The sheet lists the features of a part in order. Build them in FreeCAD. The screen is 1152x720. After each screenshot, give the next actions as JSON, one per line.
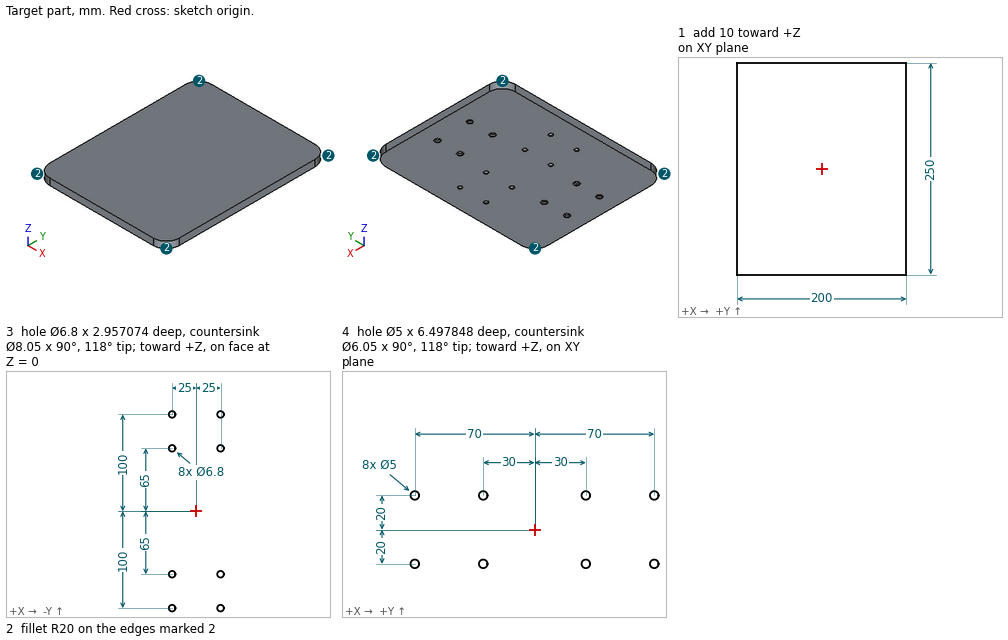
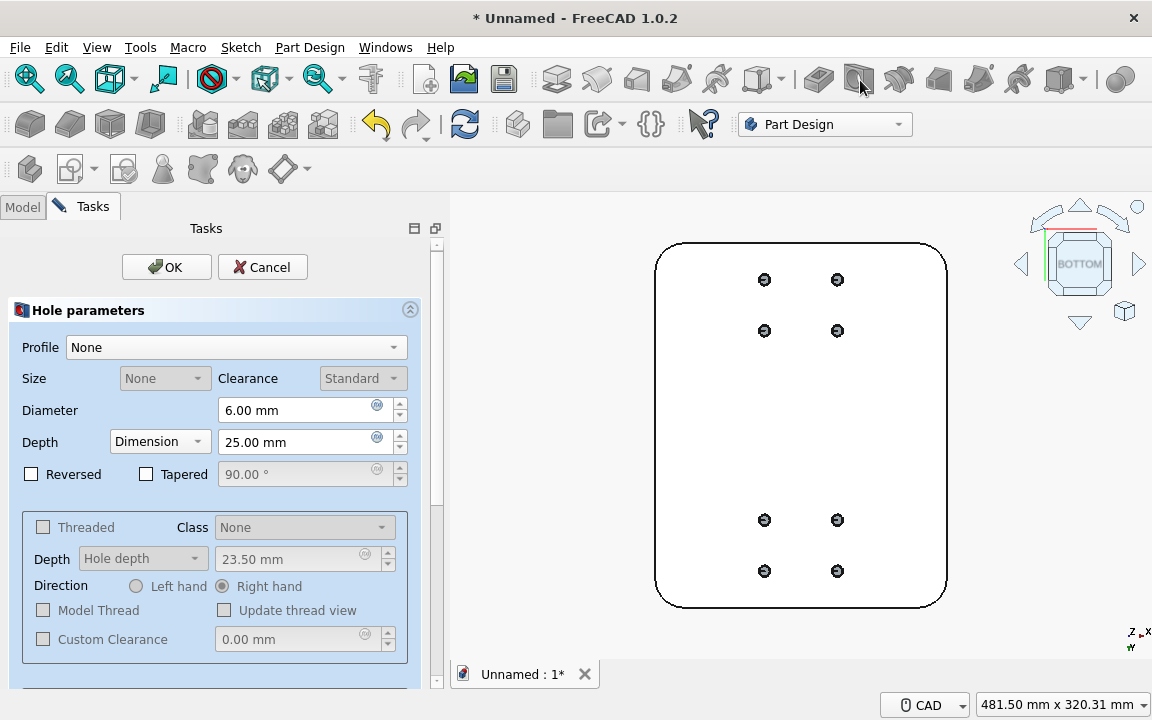
{"action": "triple_click", "coordinate": [305, 410]}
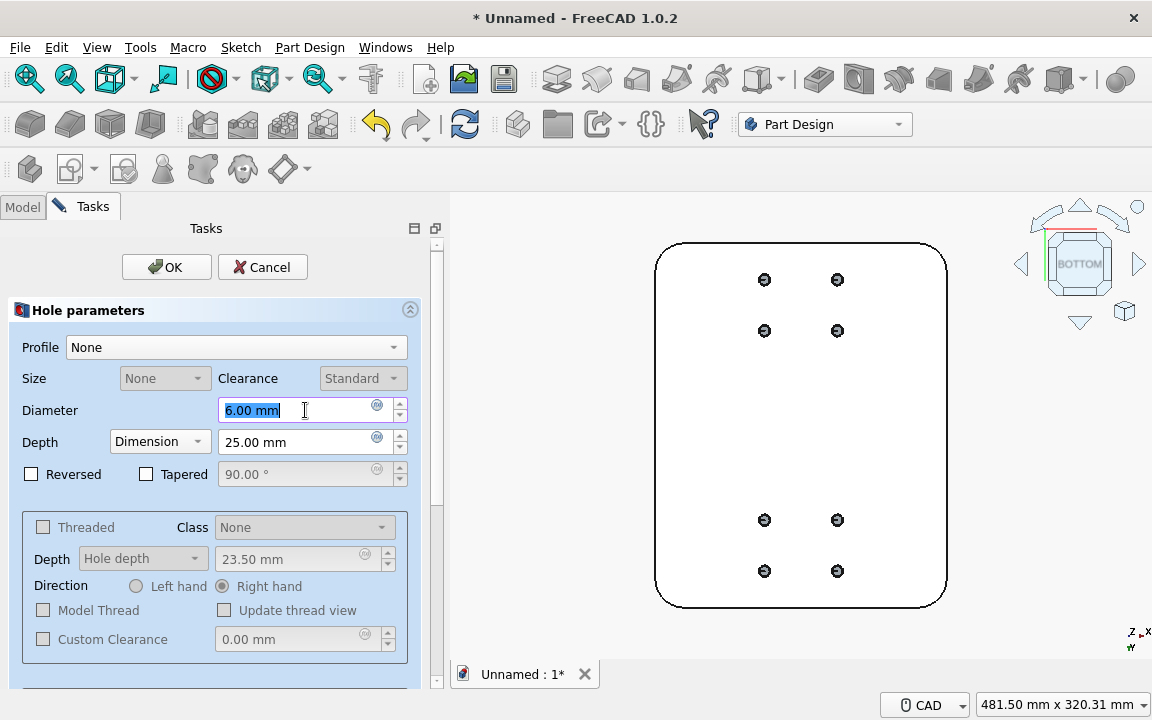
{"action": "type", "text": "5"}
{"action": "key", "text": "Tab"}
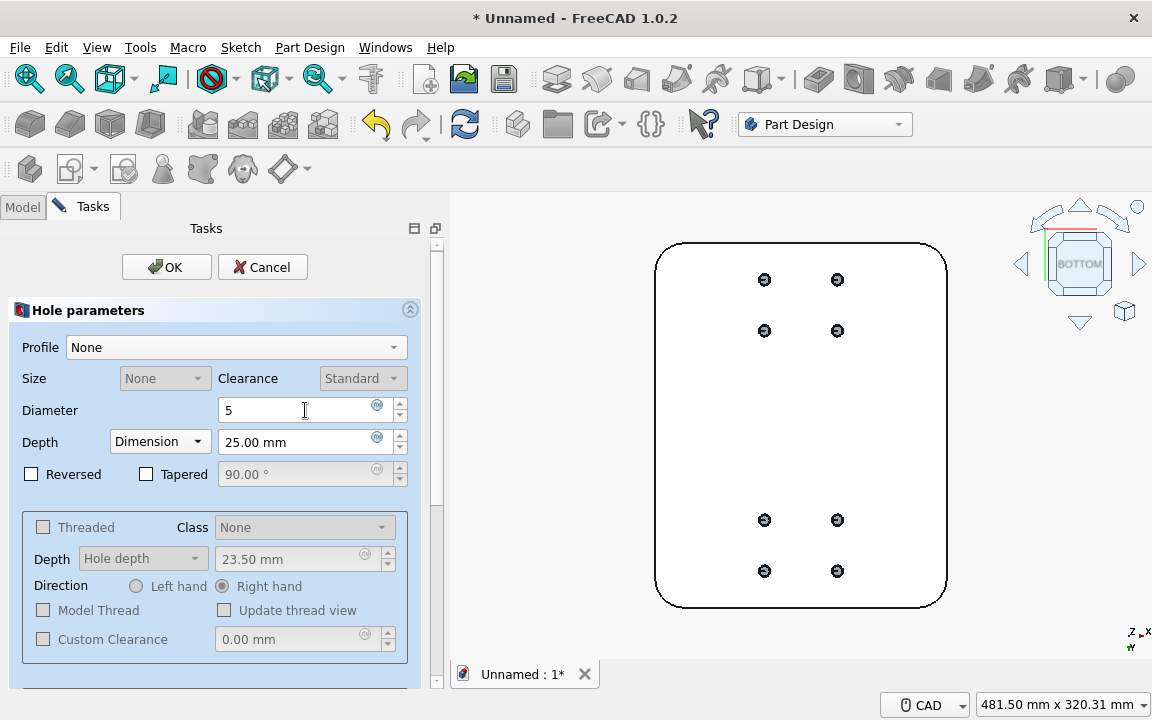
{"action": "triple_click", "coordinate": [305, 442]}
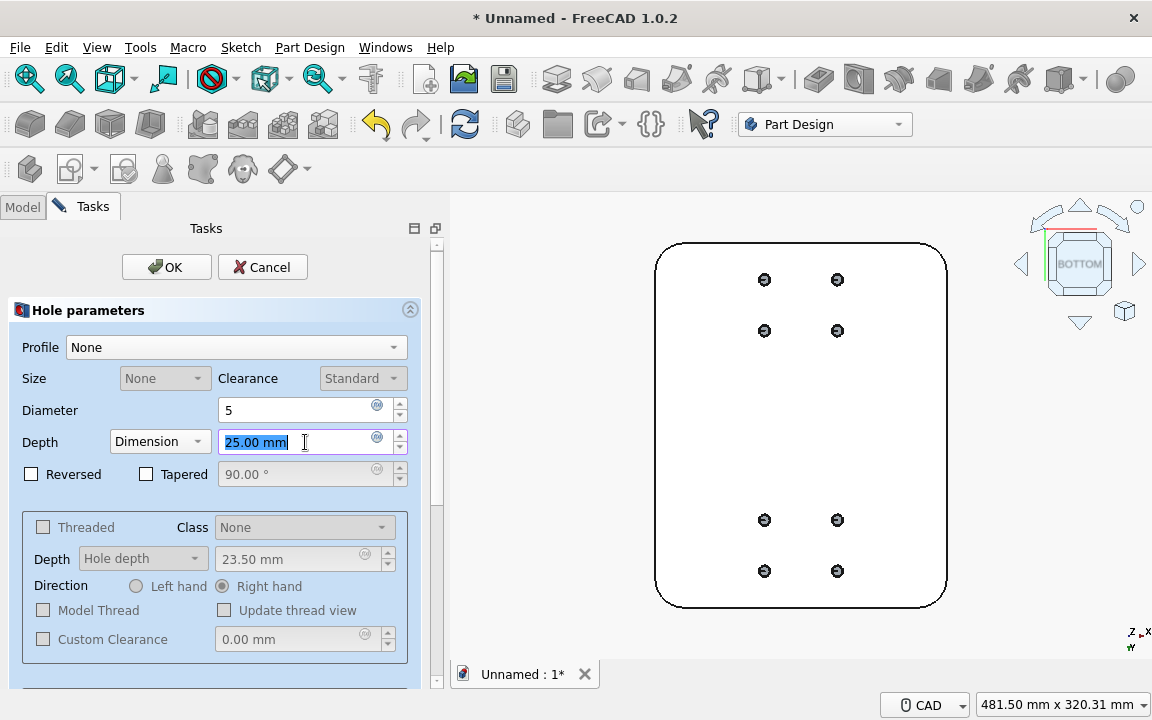
{"action": "type", "text": "6.497848"}
{"action": "key", "text": "Tab"}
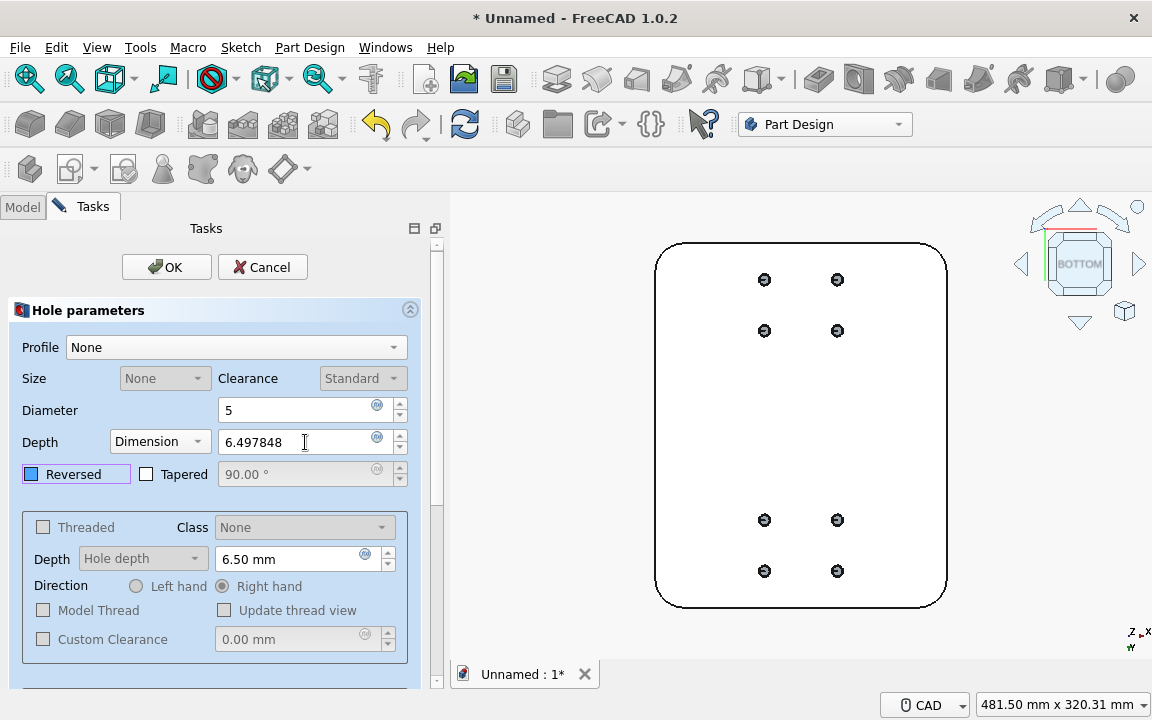
{"action": "left_click", "coordinate": [30, 474]}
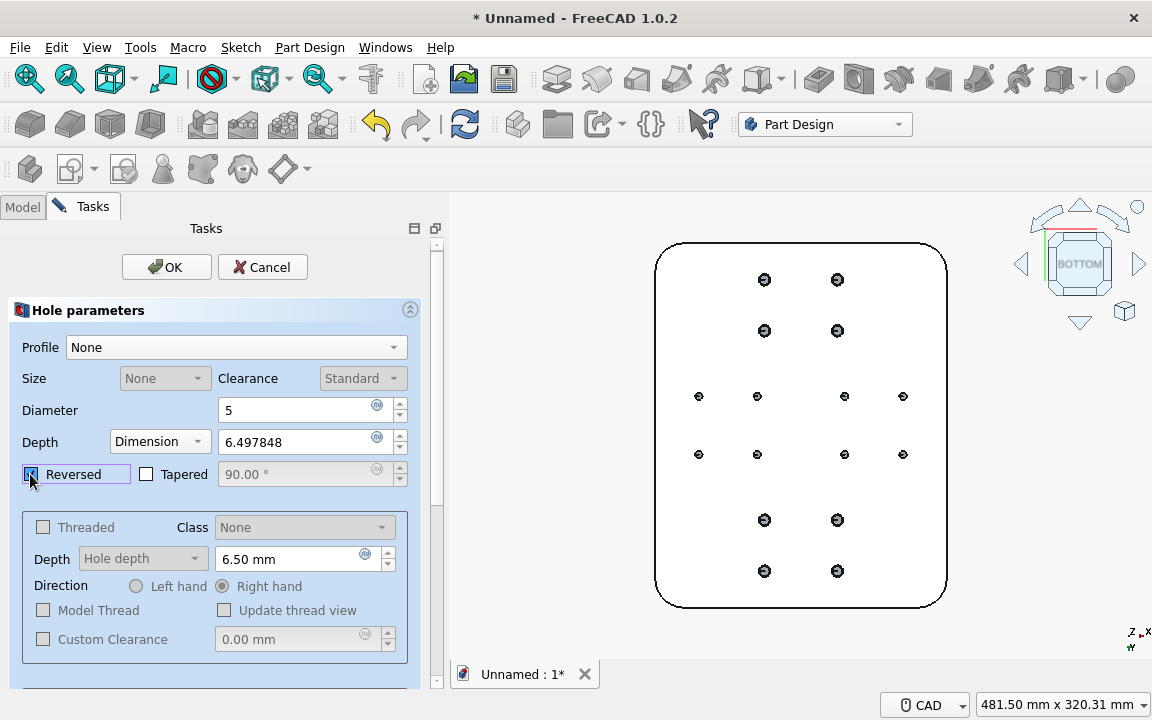
{"action": "scroll", "coordinate": [437, 463], "scroll_direction": "down", "scroll_amount": 2}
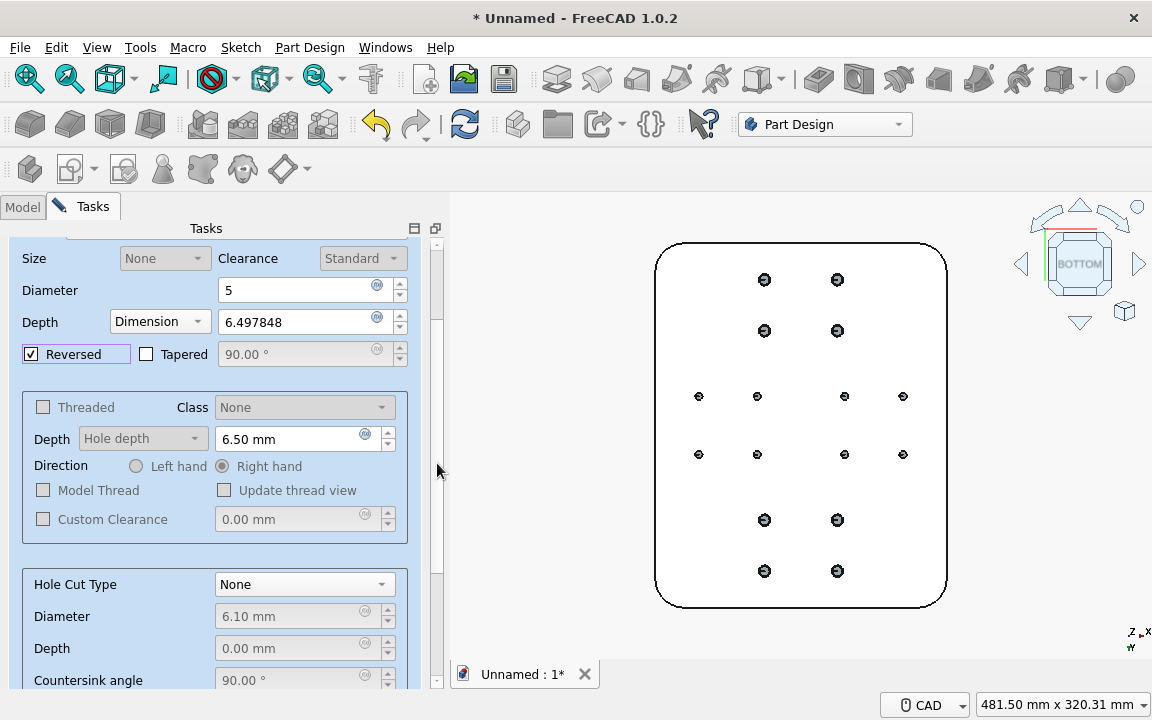
{"action": "left_click", "coordinate": [306, 584]}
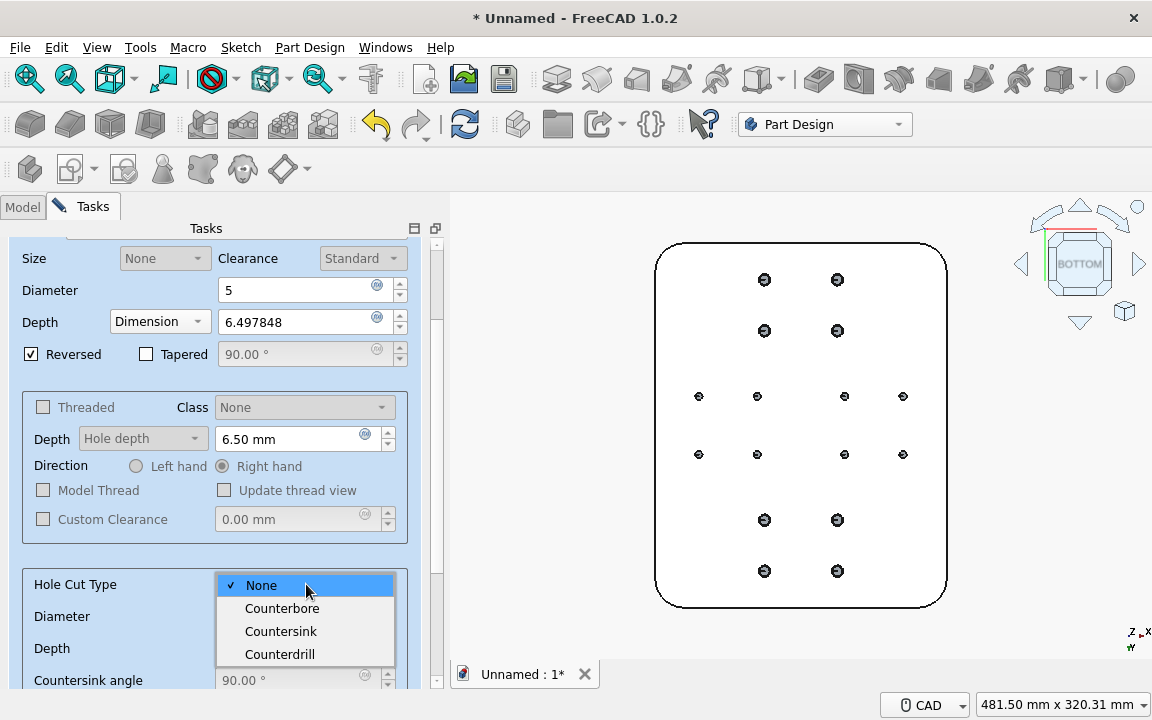
{"action": "left_click", "coordinate": [304, 632]}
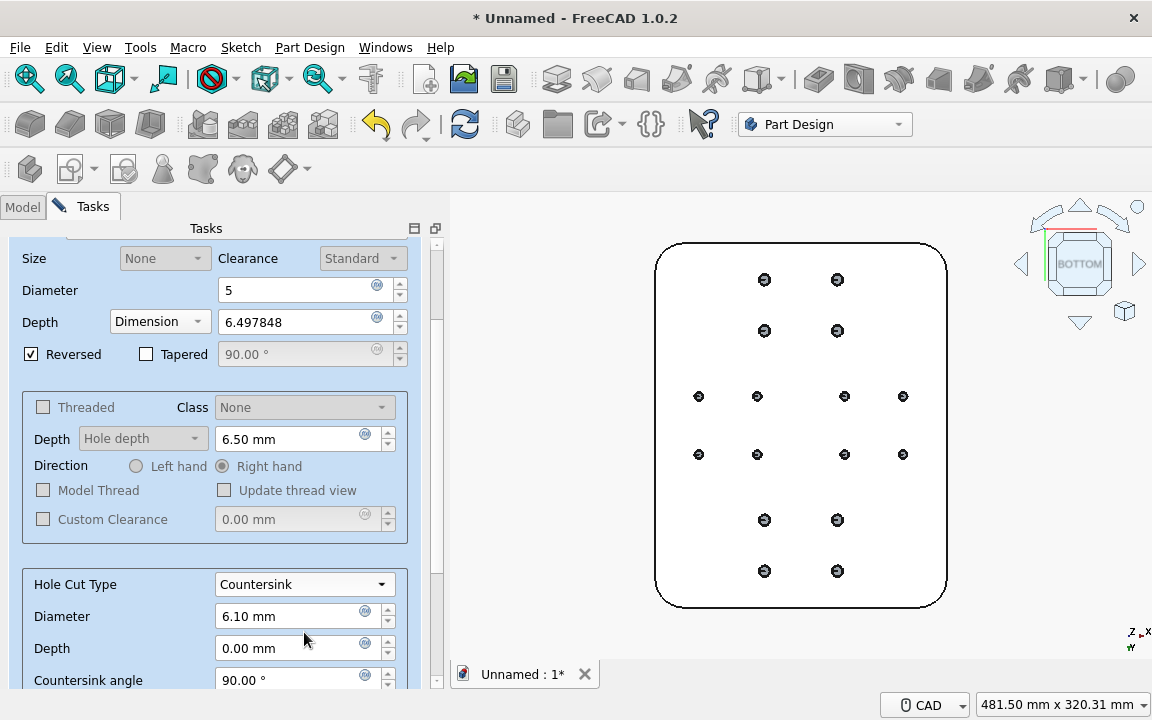
{"action": "triple_click", "coordinate": [298, 616]}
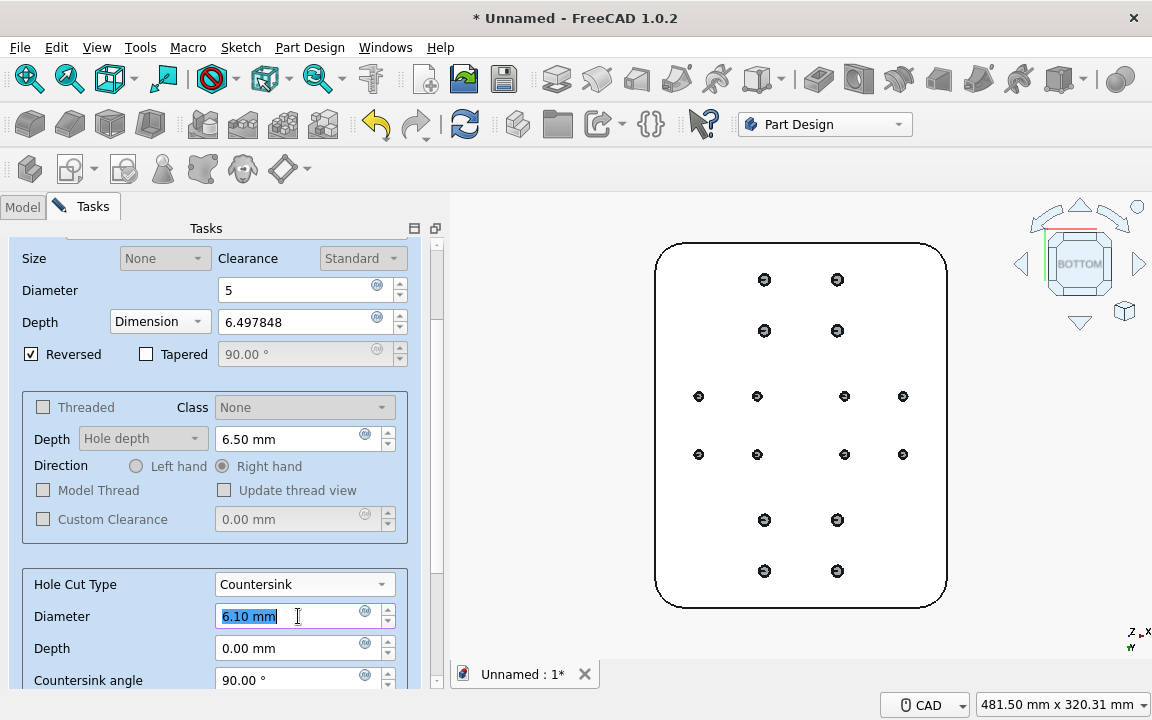
{"action": "type", "text": "6.05"}
{"action": "key", "text": "Tab"}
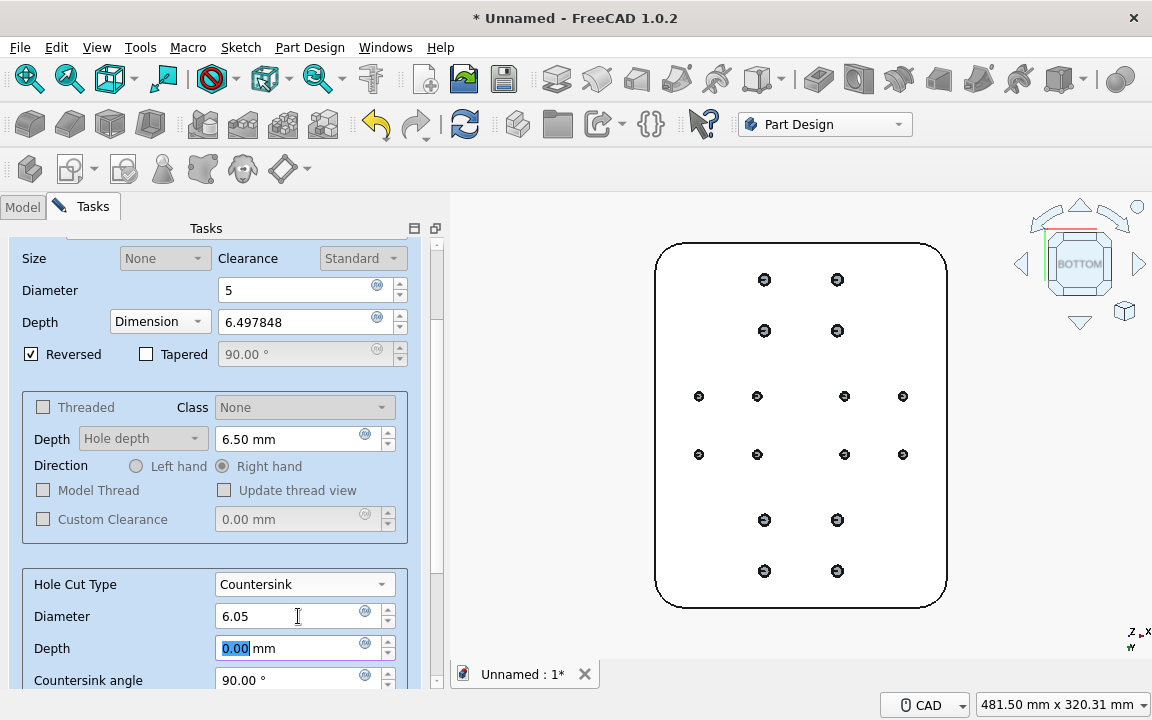
{"action": "scroll", "coordinate": [437, 463], "scroll_direction": "up", "scroll_amount": 3}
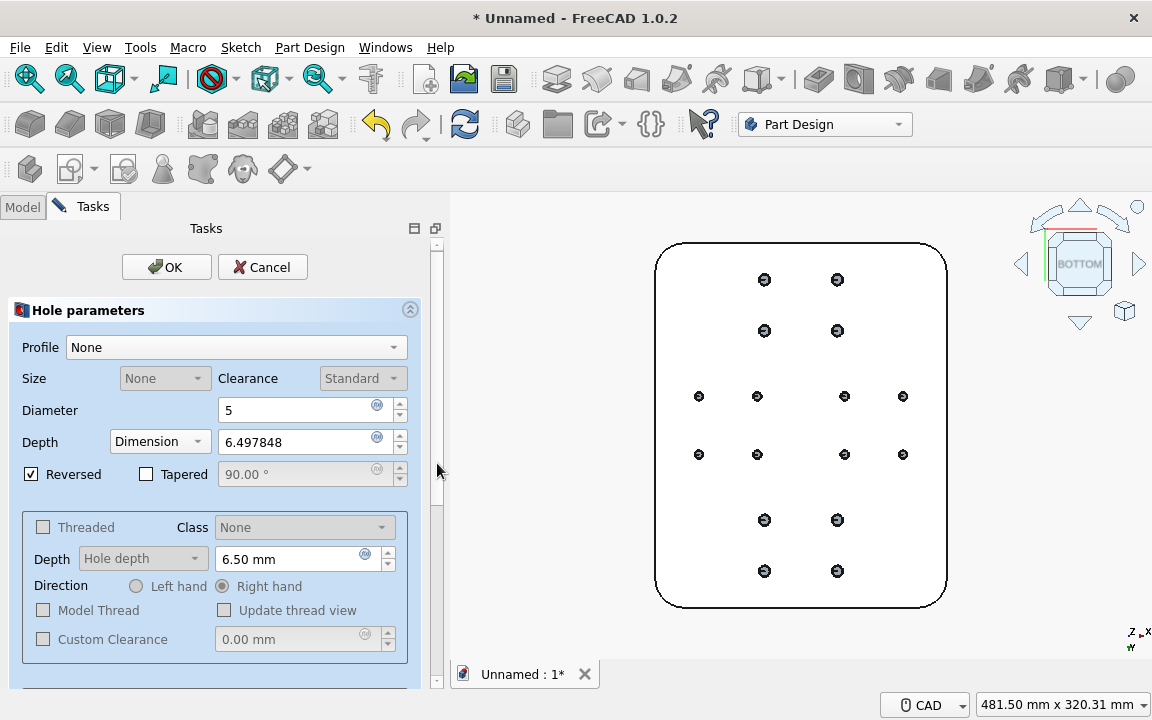
{"action": "left_click", "coordinate": [167, 267]}